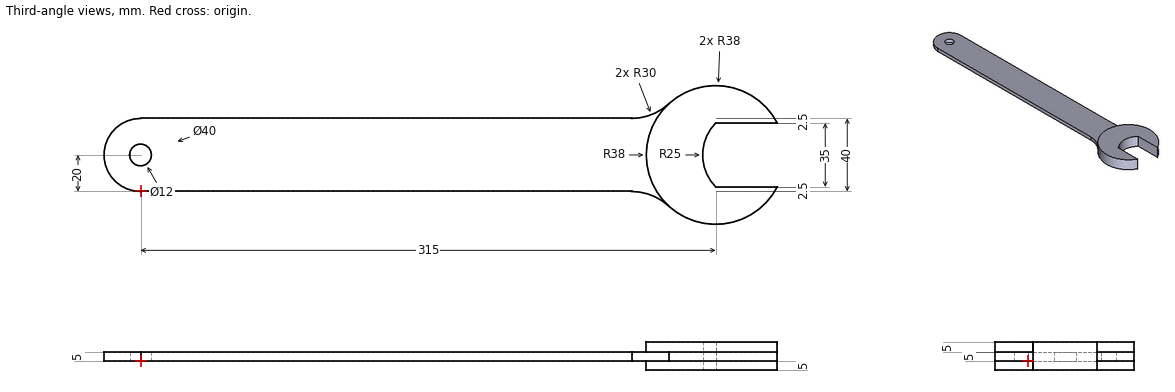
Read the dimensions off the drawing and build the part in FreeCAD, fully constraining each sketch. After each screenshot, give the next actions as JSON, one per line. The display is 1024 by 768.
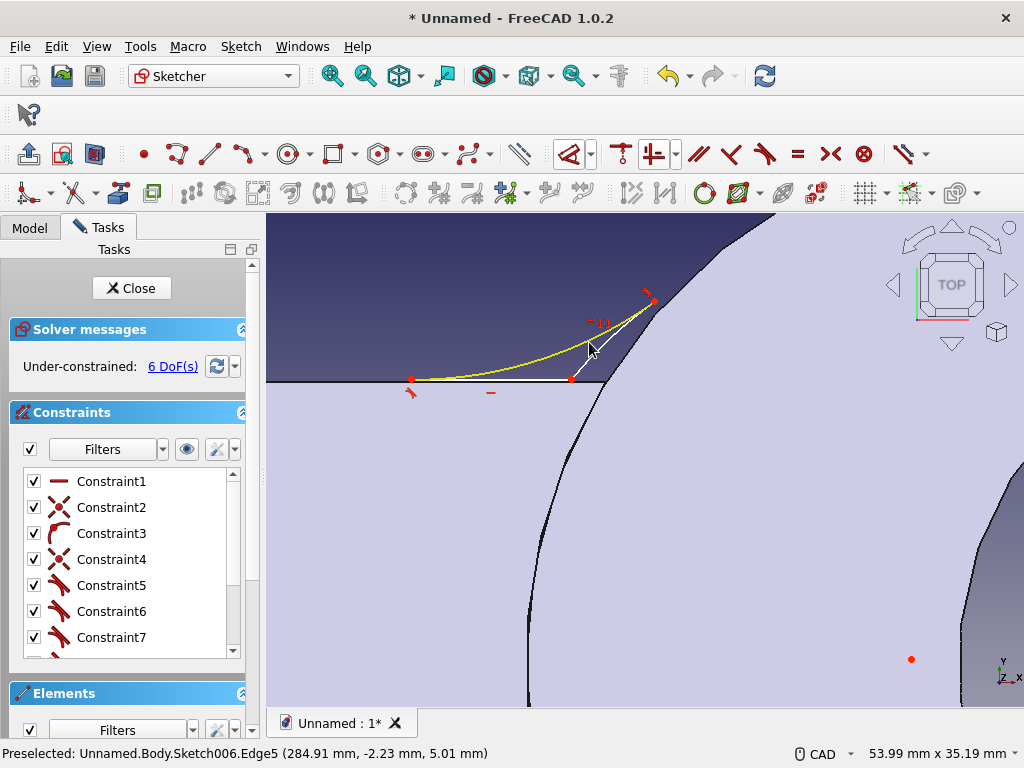
{"action": "left_click", "coordinate": [588, 341]}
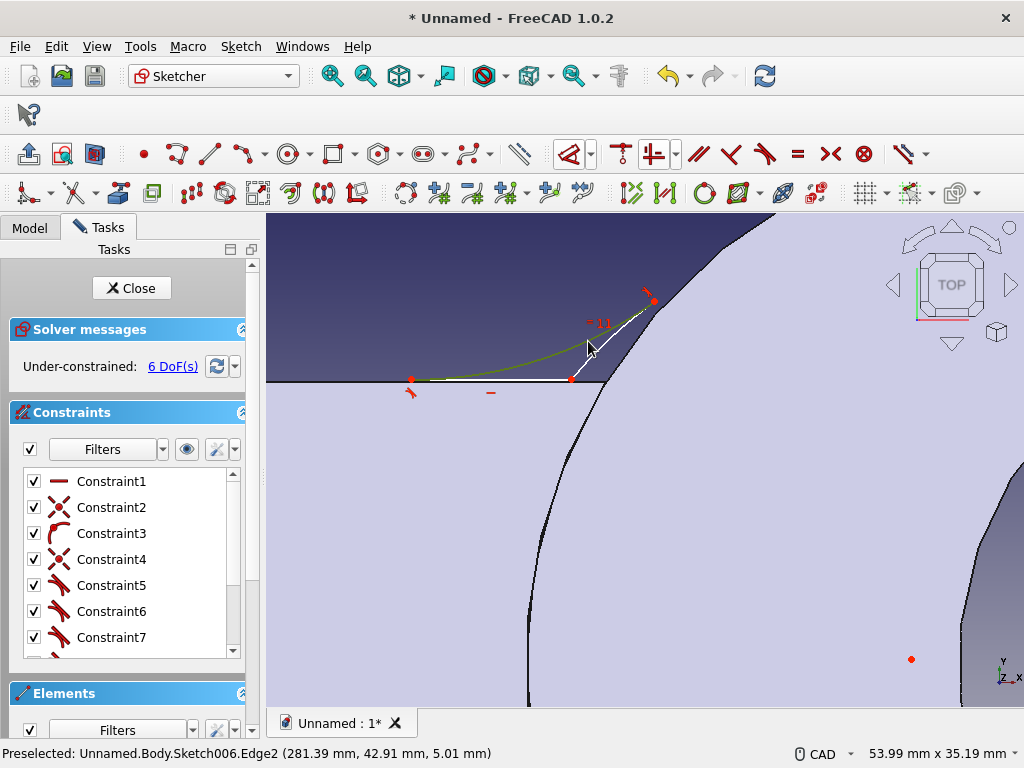
{"action": "scroll", "coordinate": [589, 342], "scroll_direction": "down", "scroll_amount": 5}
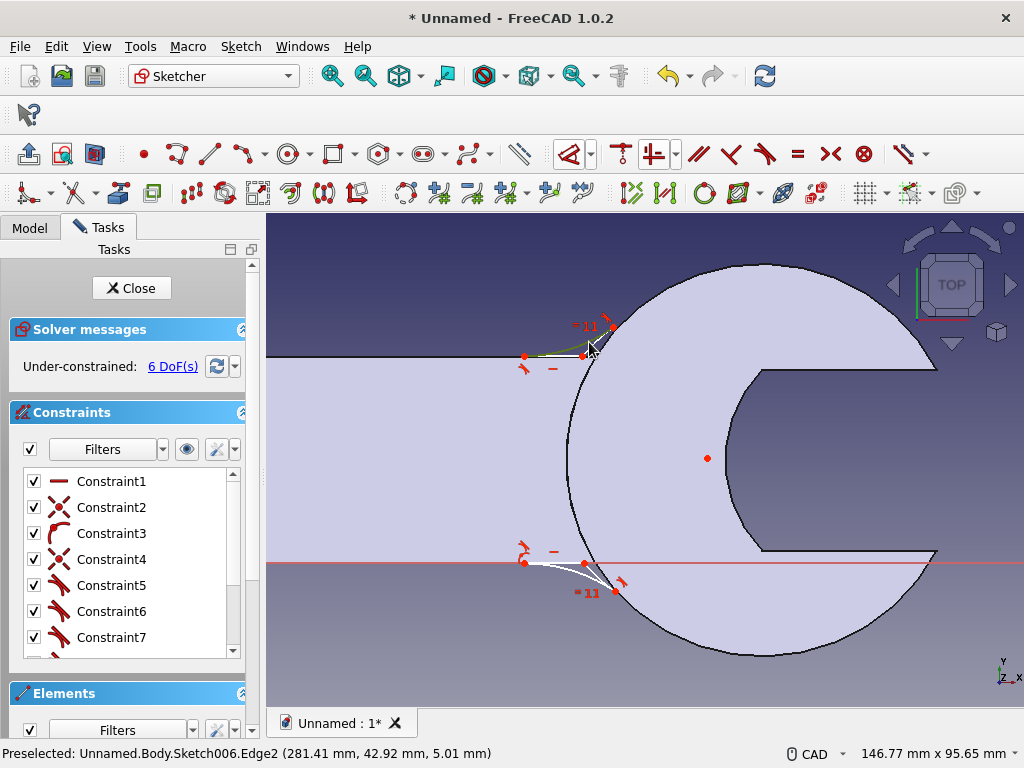
{"action": "scroll", "coordinate": [590, 578], "scroll_direction": "up", "scroll_amount": 5}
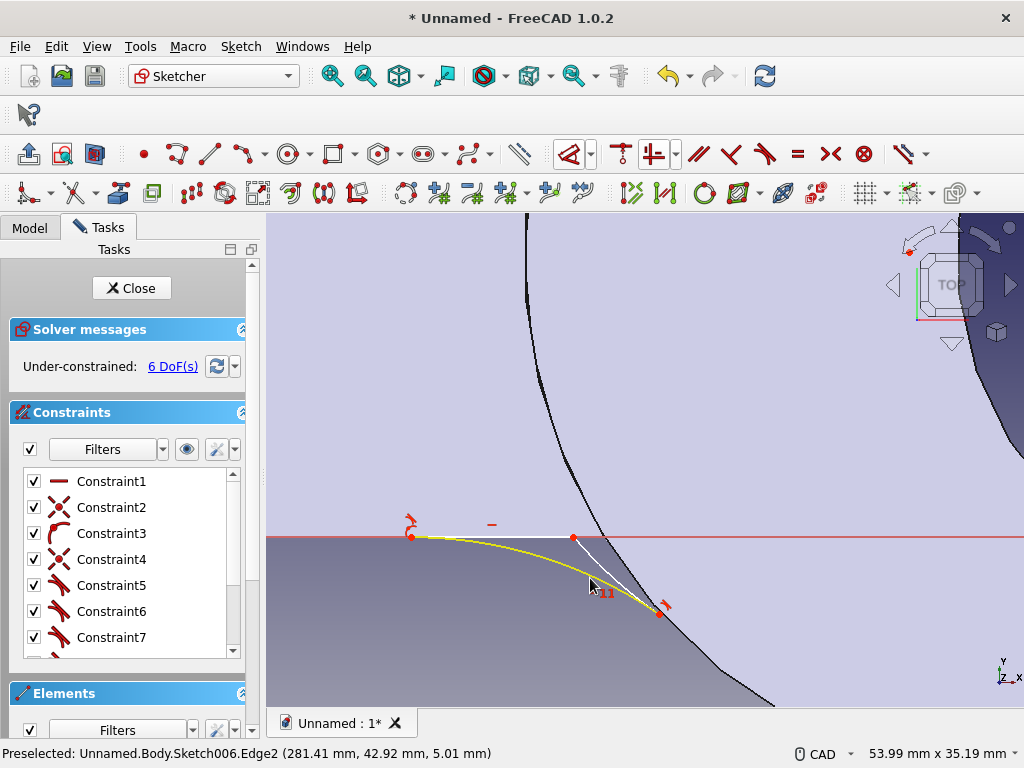
{"action": "left_click", "coordinate": [591, 576]}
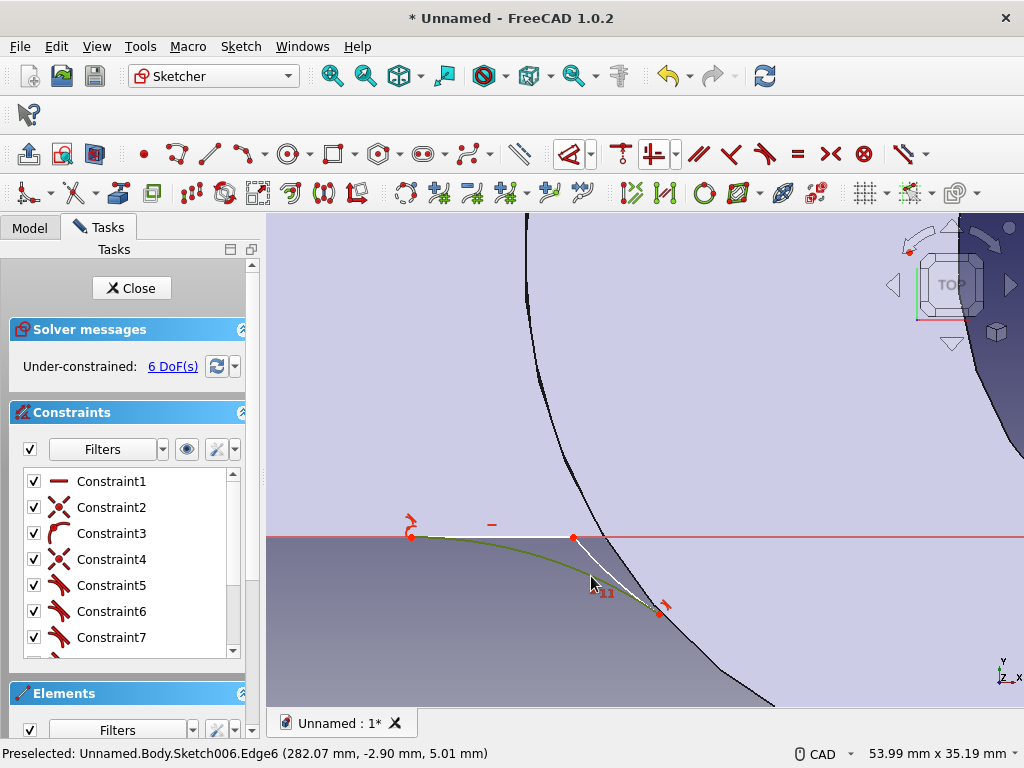
{"action": "left_click", "coordinate": [798, 154]}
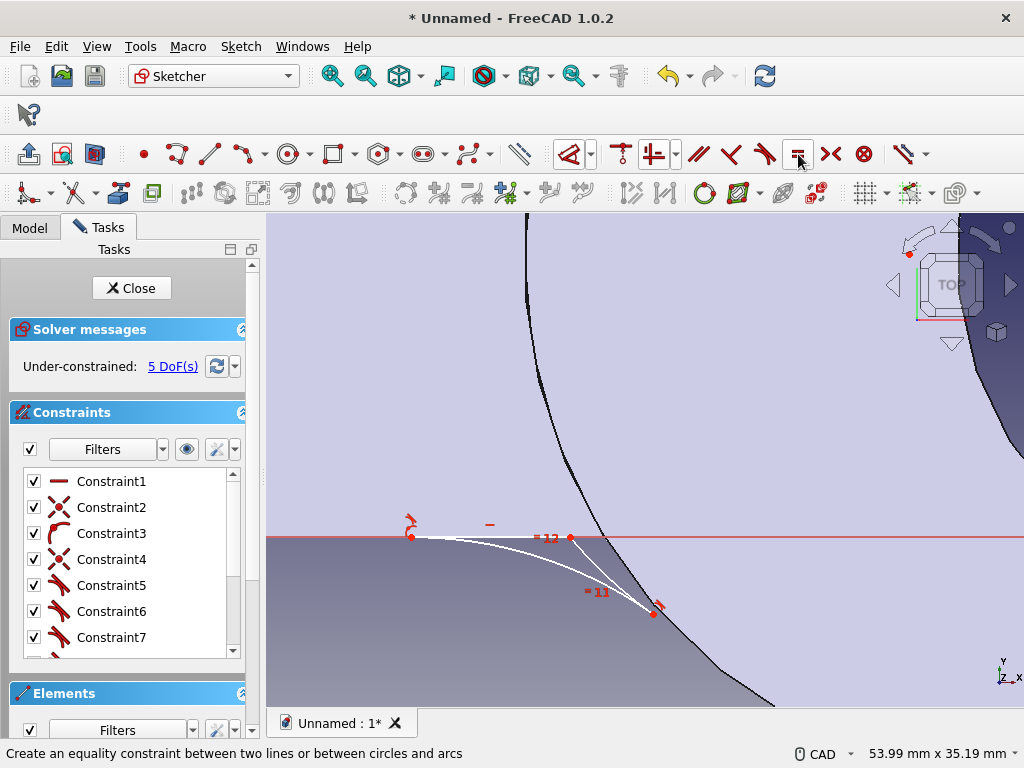
{"action": "scroll", "coordinate": [590, 579], "scroll_direction": "down", "scroll_amount": 5}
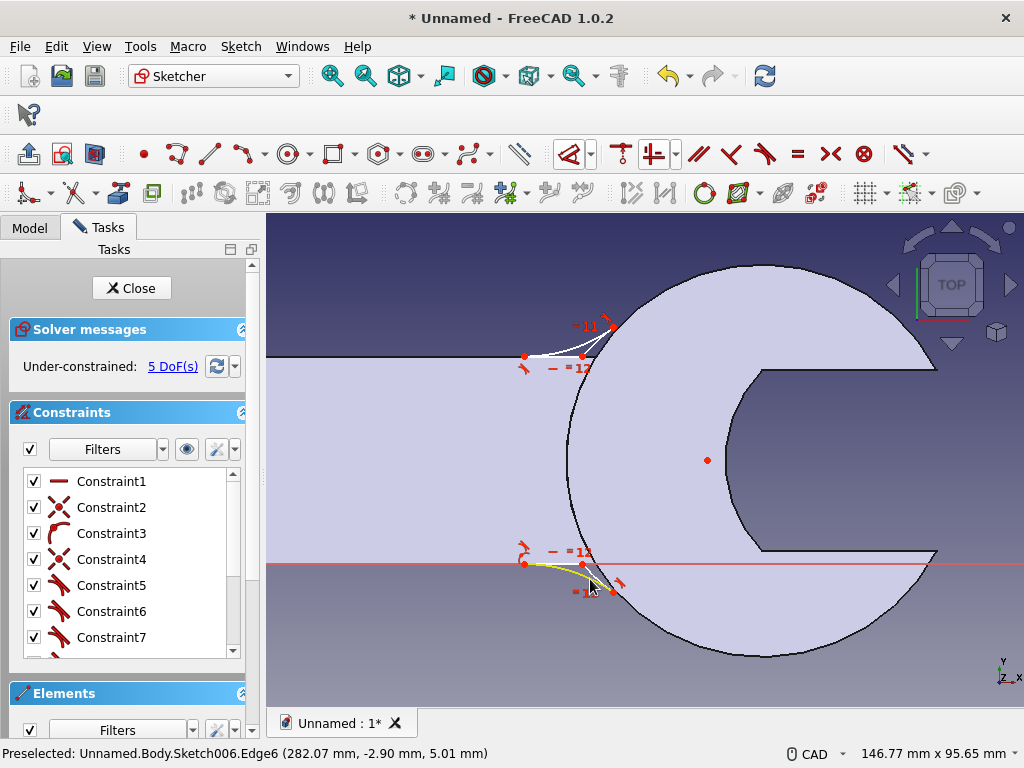
{"action": "scroll", "coordinate": [589, 342], "scroll_direction": "up", "scroll_amount": 6}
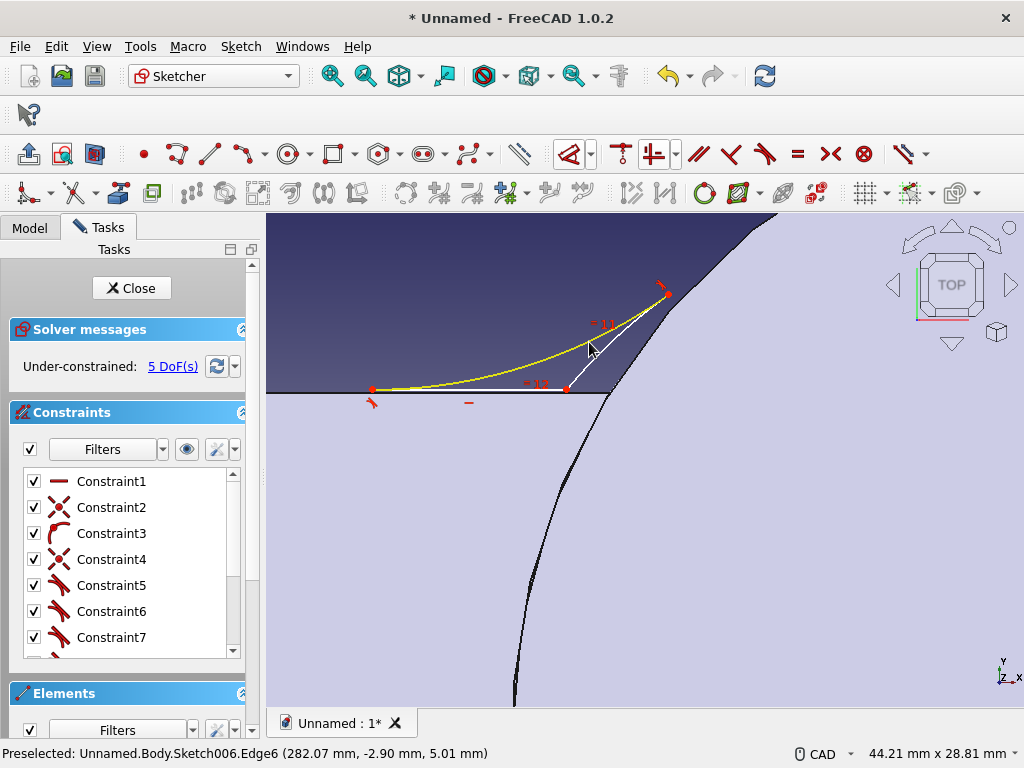
{"action": "left_click", "coordinate": [587, 343]}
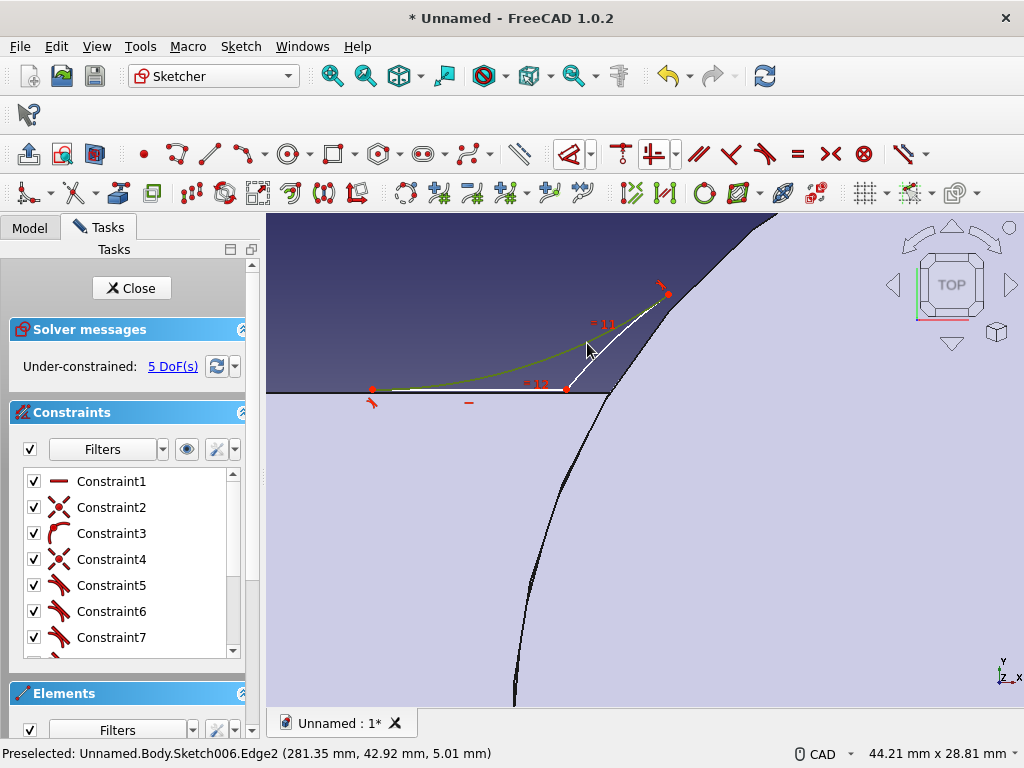
{"action": "left_click", "coordinate": [590, 154]}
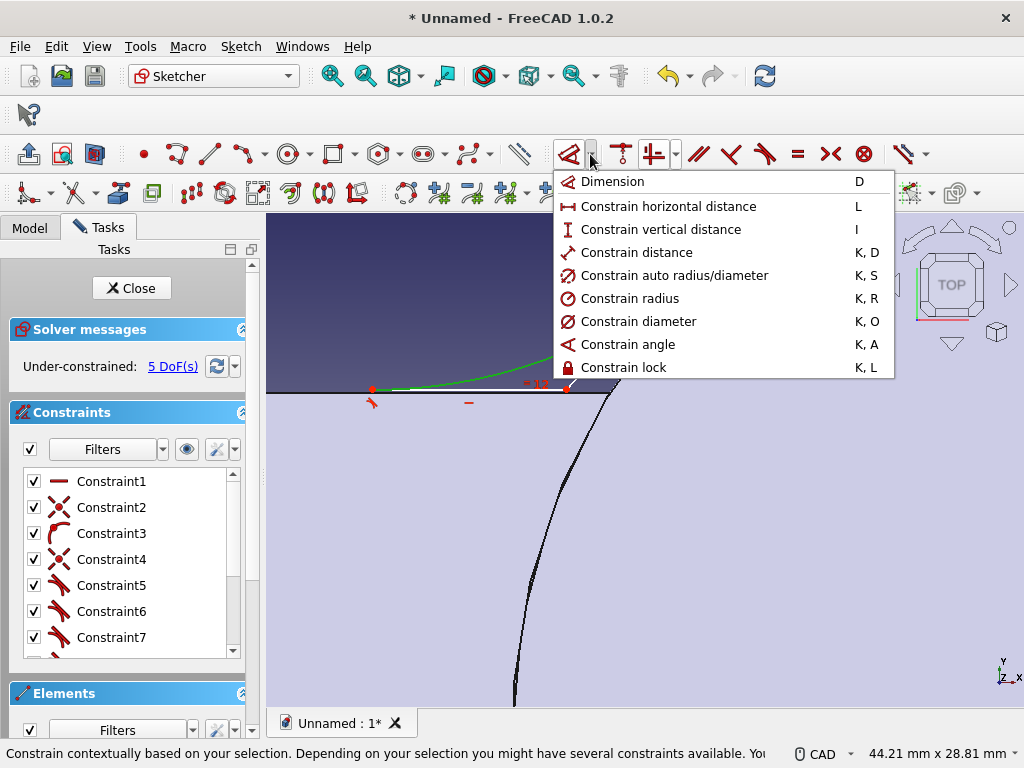
{"action": "left_click", "coordinate": [724, 298]}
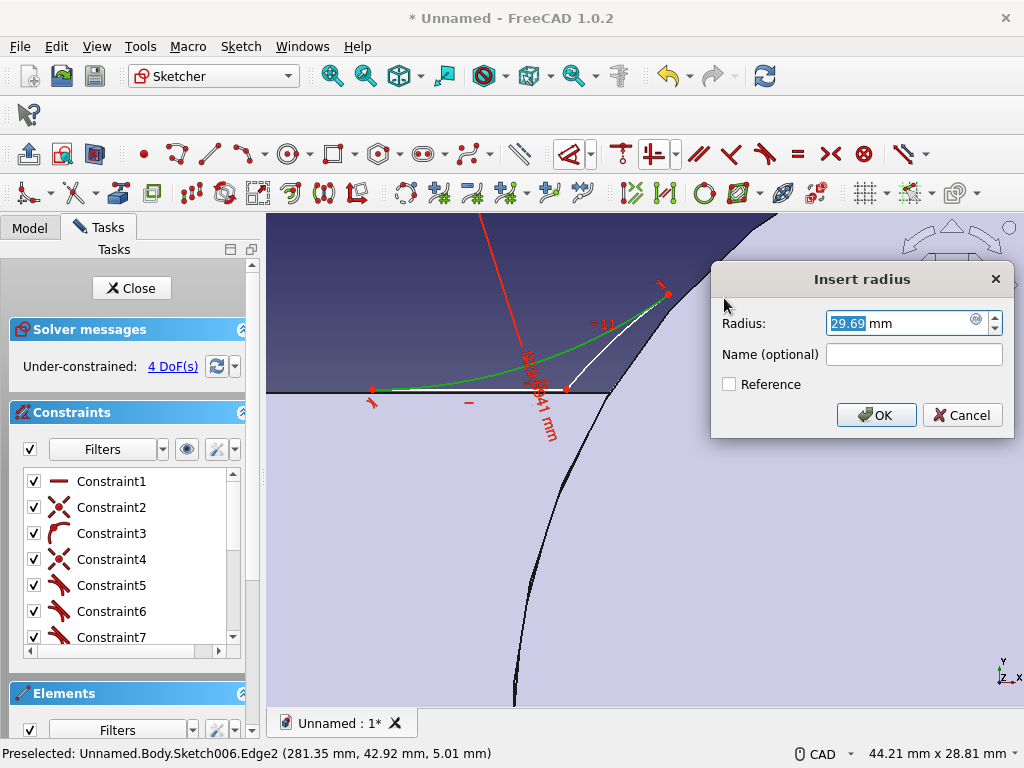
{"action": "type", "text": "30"}
{"action": "key", "text": "Return"}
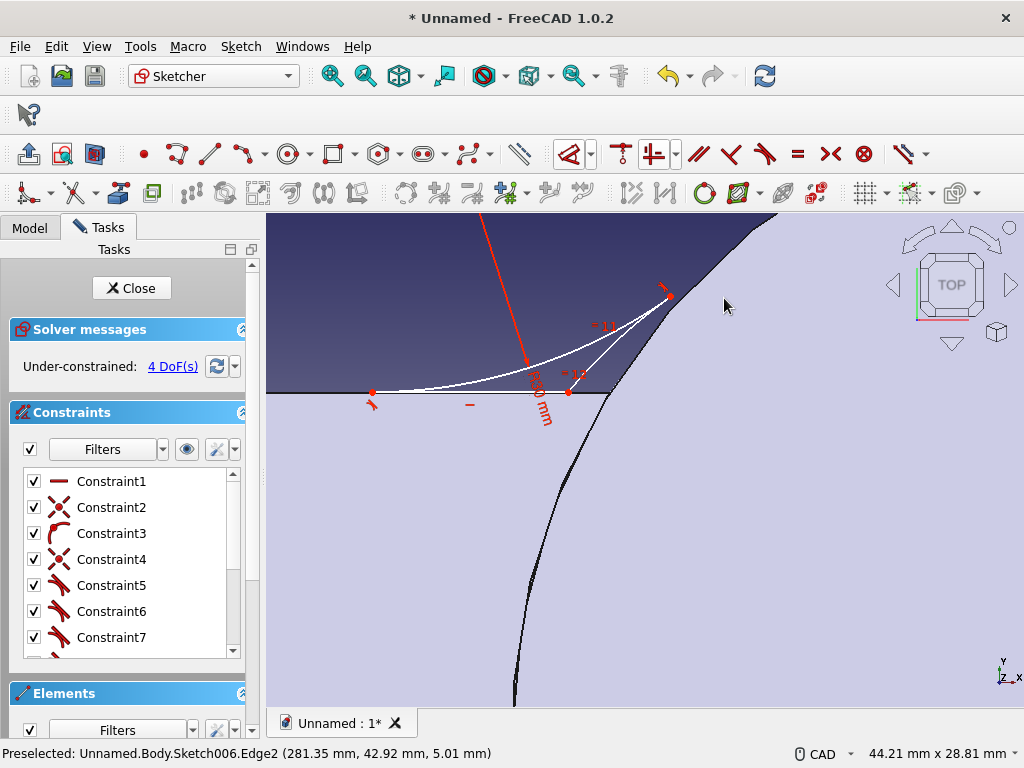
{"action": "left_click", "coordinate": [596, 361]}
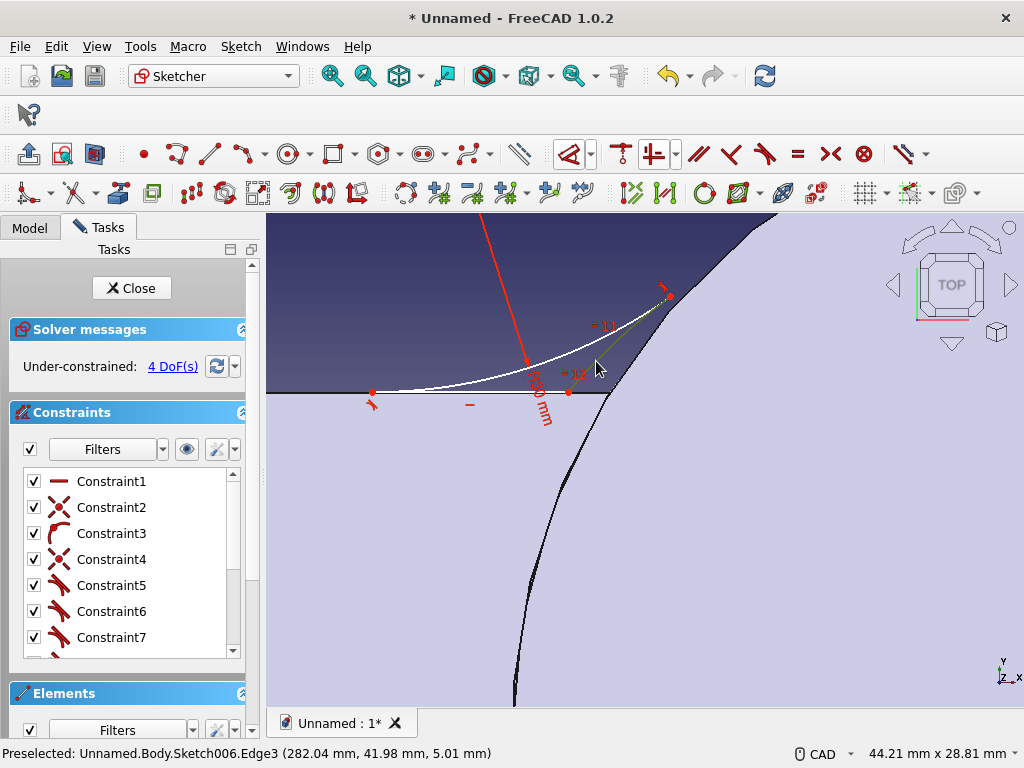
{"action": "key", "text": "k r"}